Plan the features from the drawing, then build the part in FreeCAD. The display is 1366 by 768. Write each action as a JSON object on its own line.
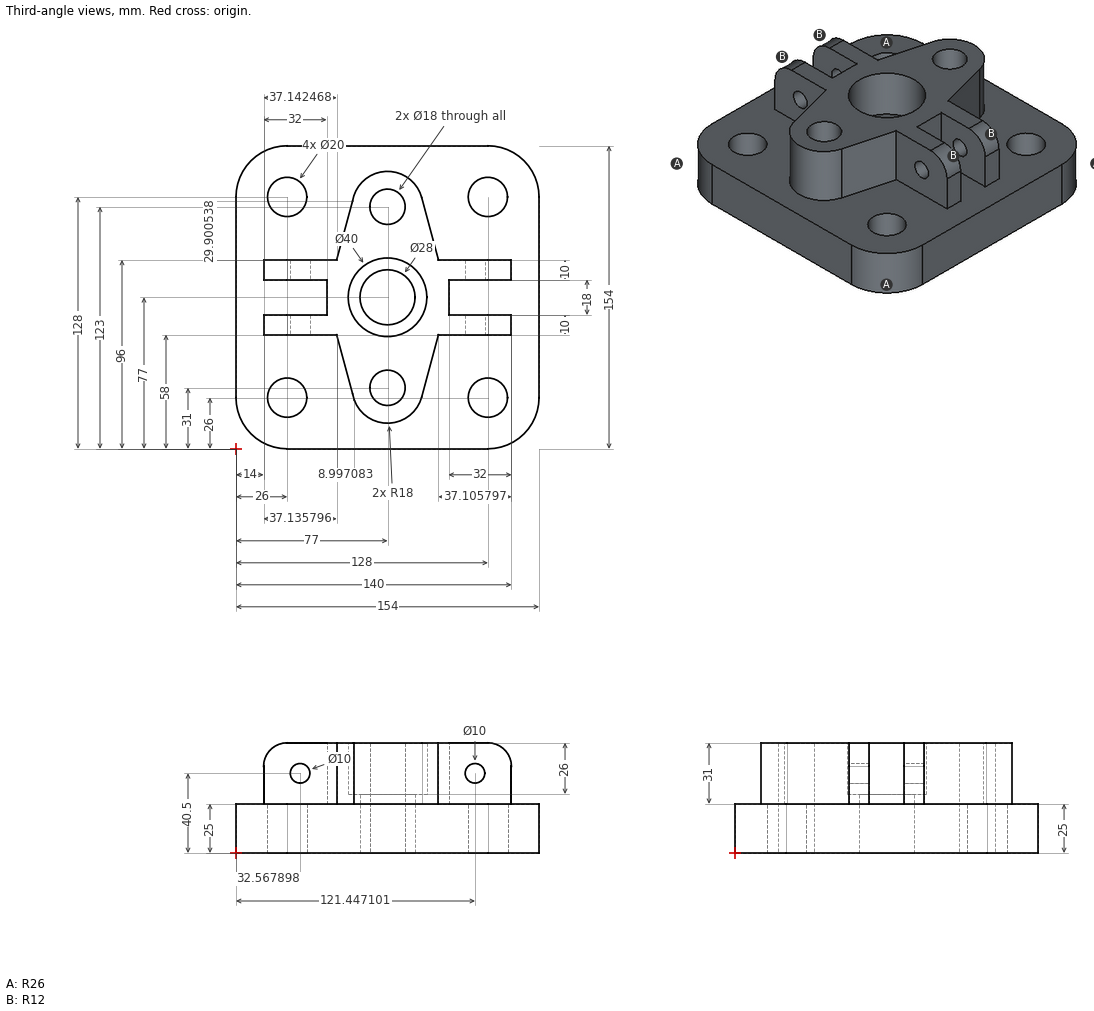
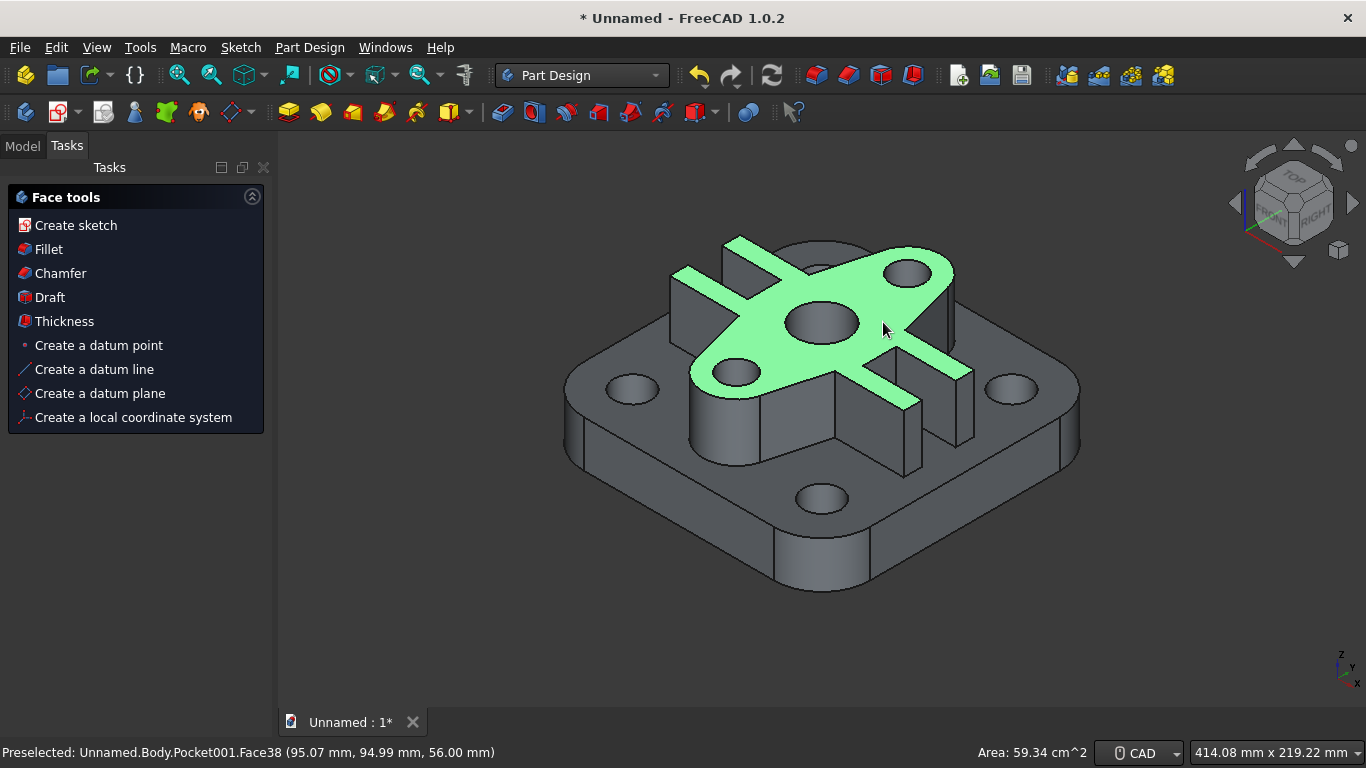
{"action": "left_click", "coordinate": [58, 112]}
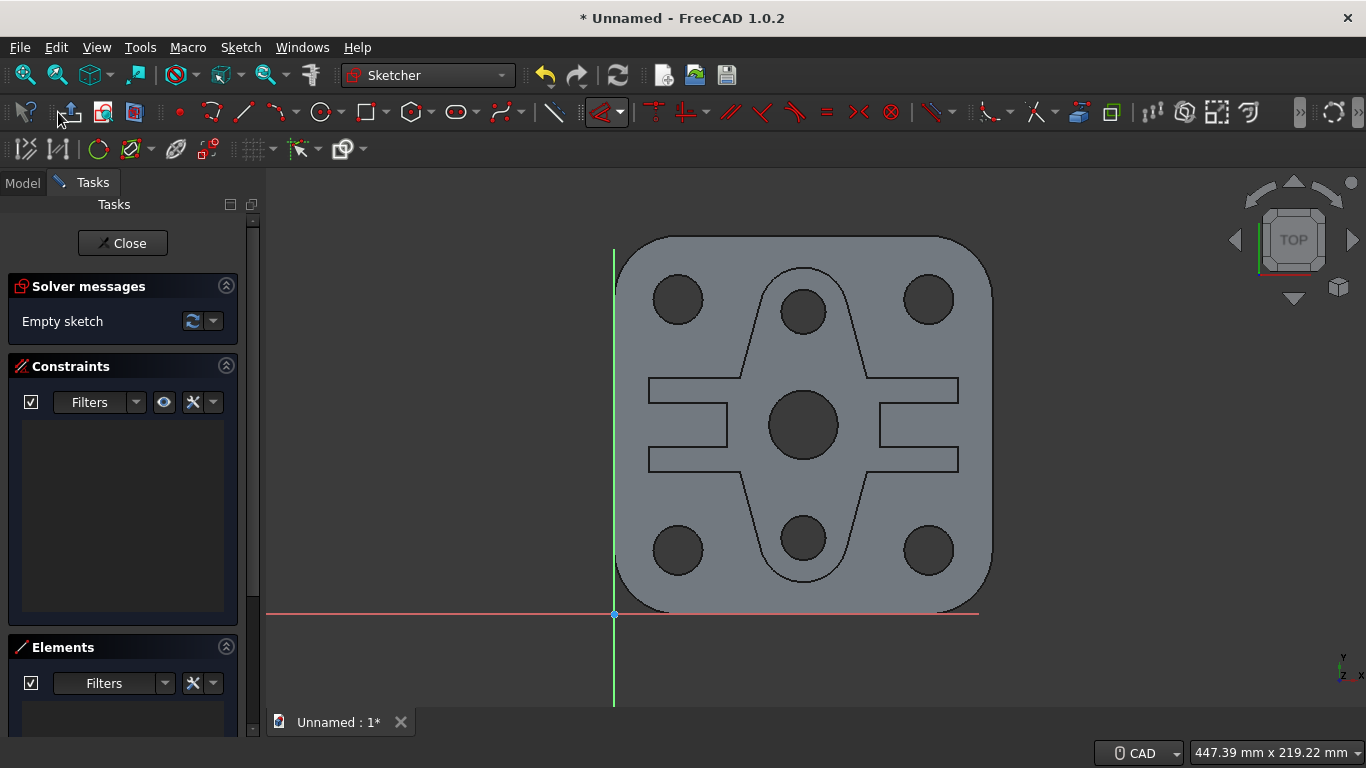
{"action": "scroll", "coordinate": [705, 612], "scroll_direction": "up", "scroll_amount": 2}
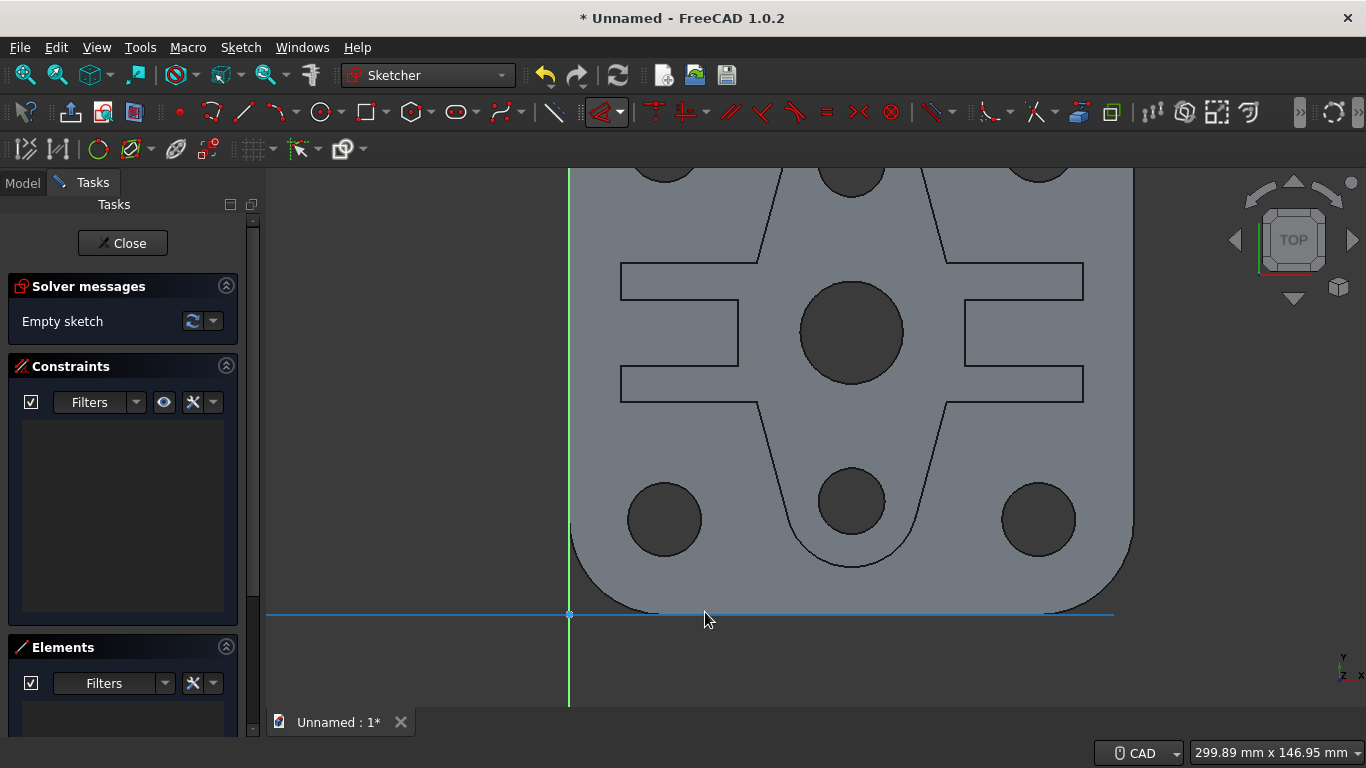
{"action": "left_click", "coordinate": [322, 112]}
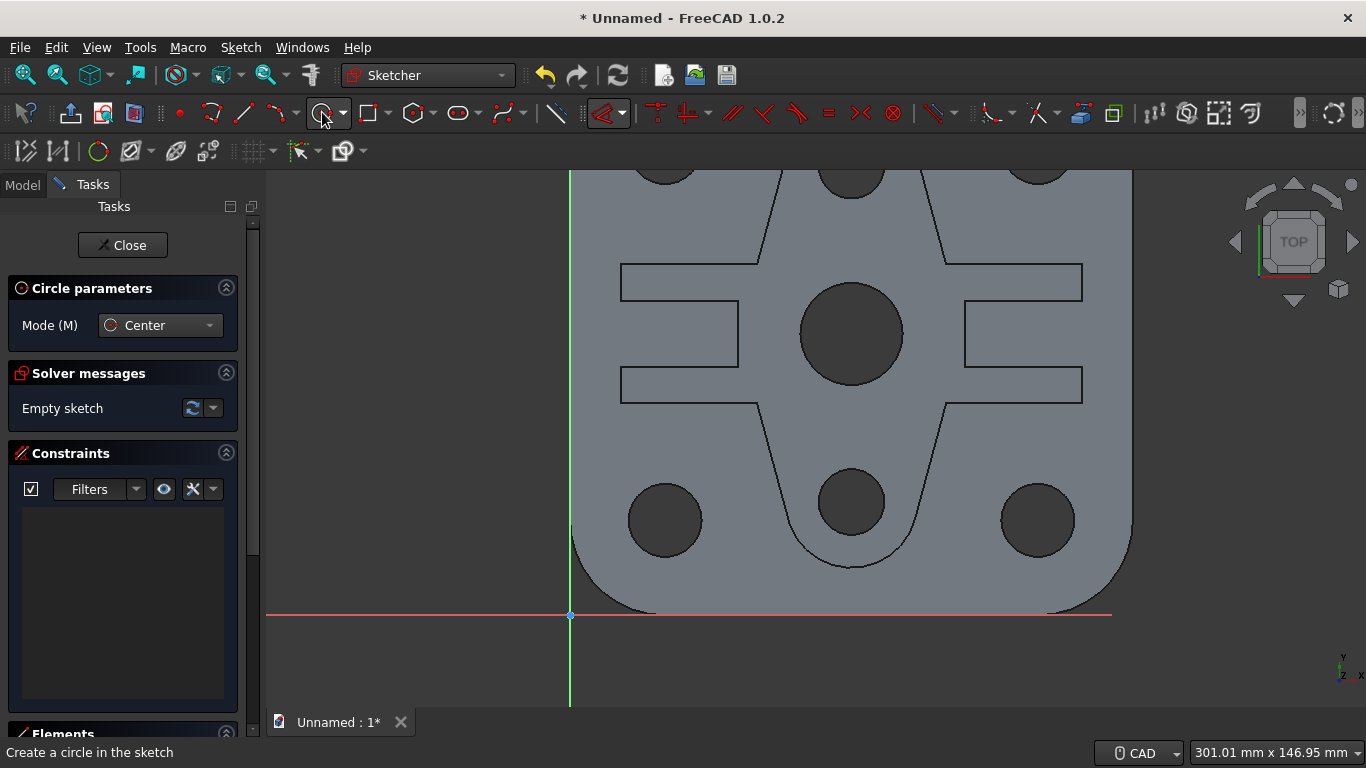
{"action": "left_click", "coordinate": [852, 334]}
{"action": "left_click", "coordinate": [903, 282]}
{"action": "key", "text": "Escape"}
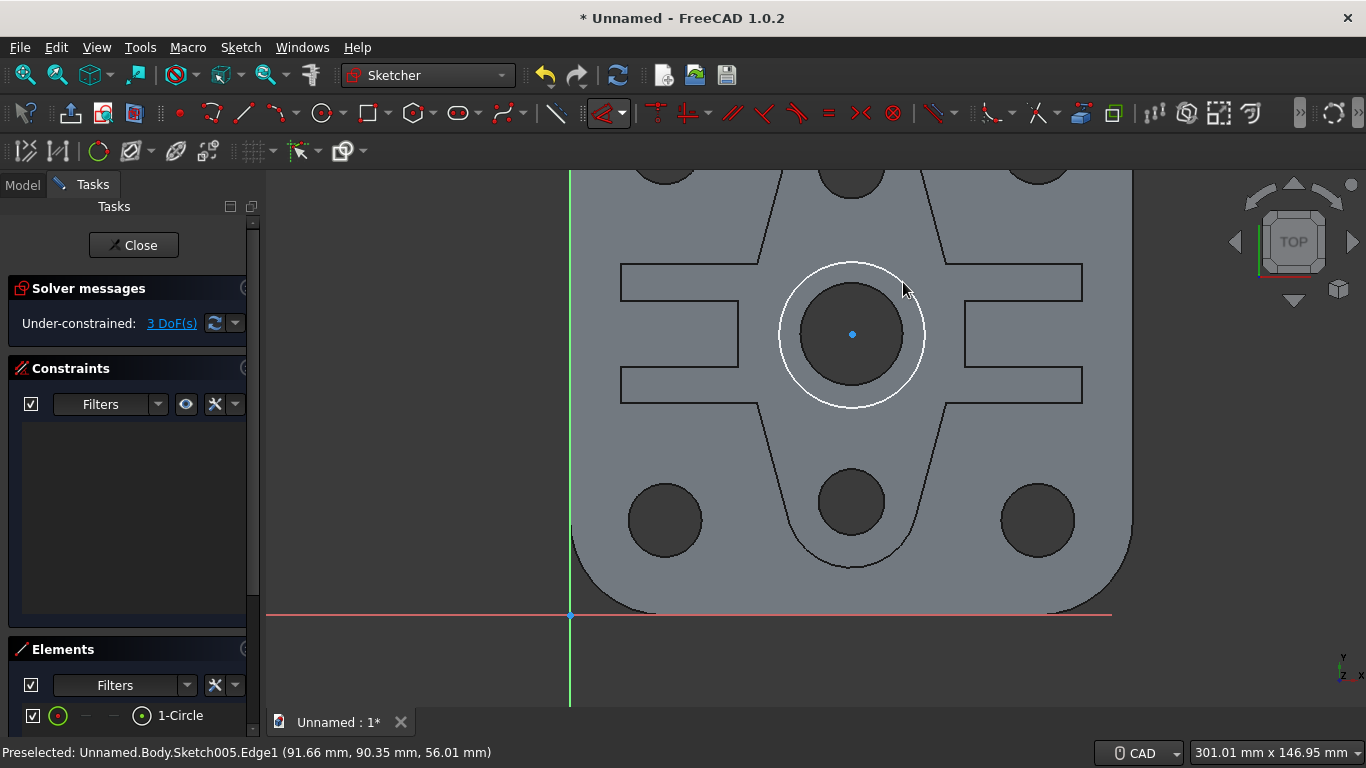
{"action": "left_click", "coordinate": [903, 283]}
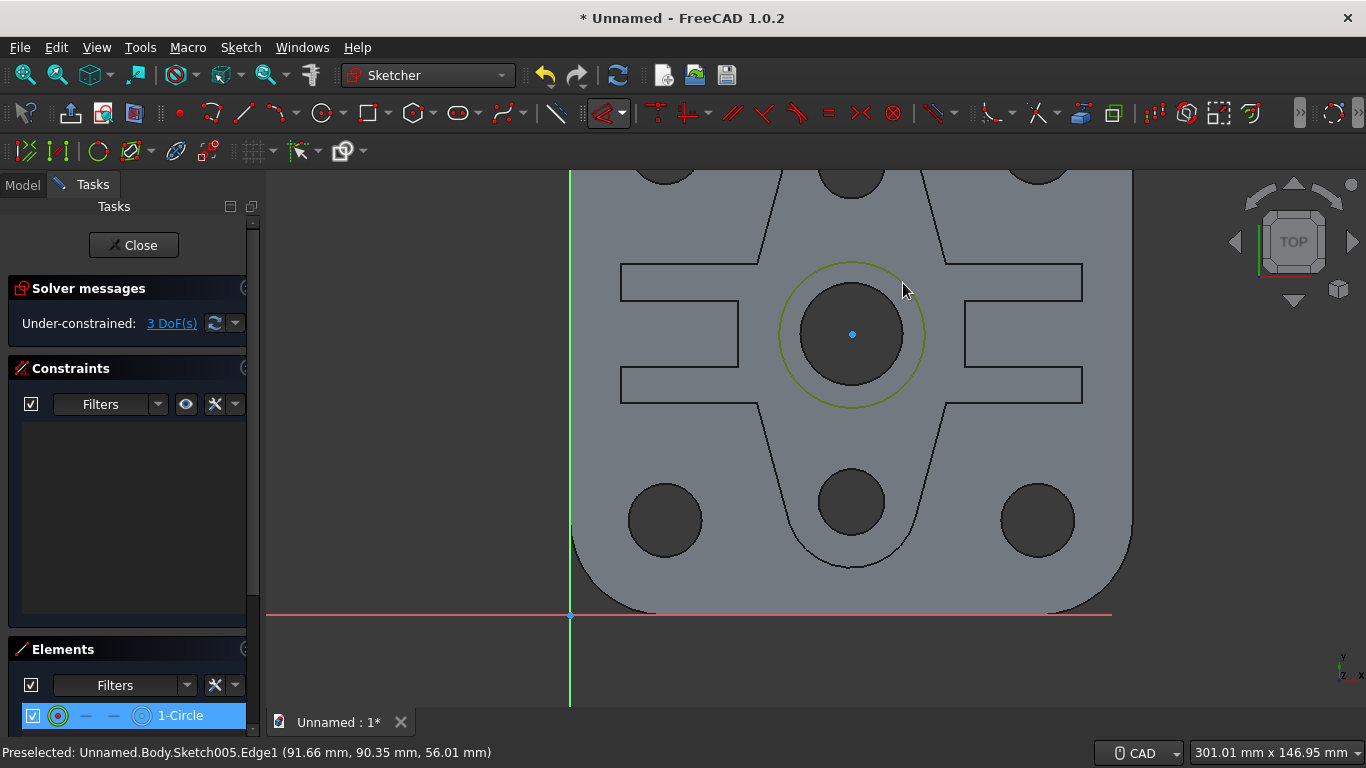
{"action": "left_click", "coordinate": [624, 114]}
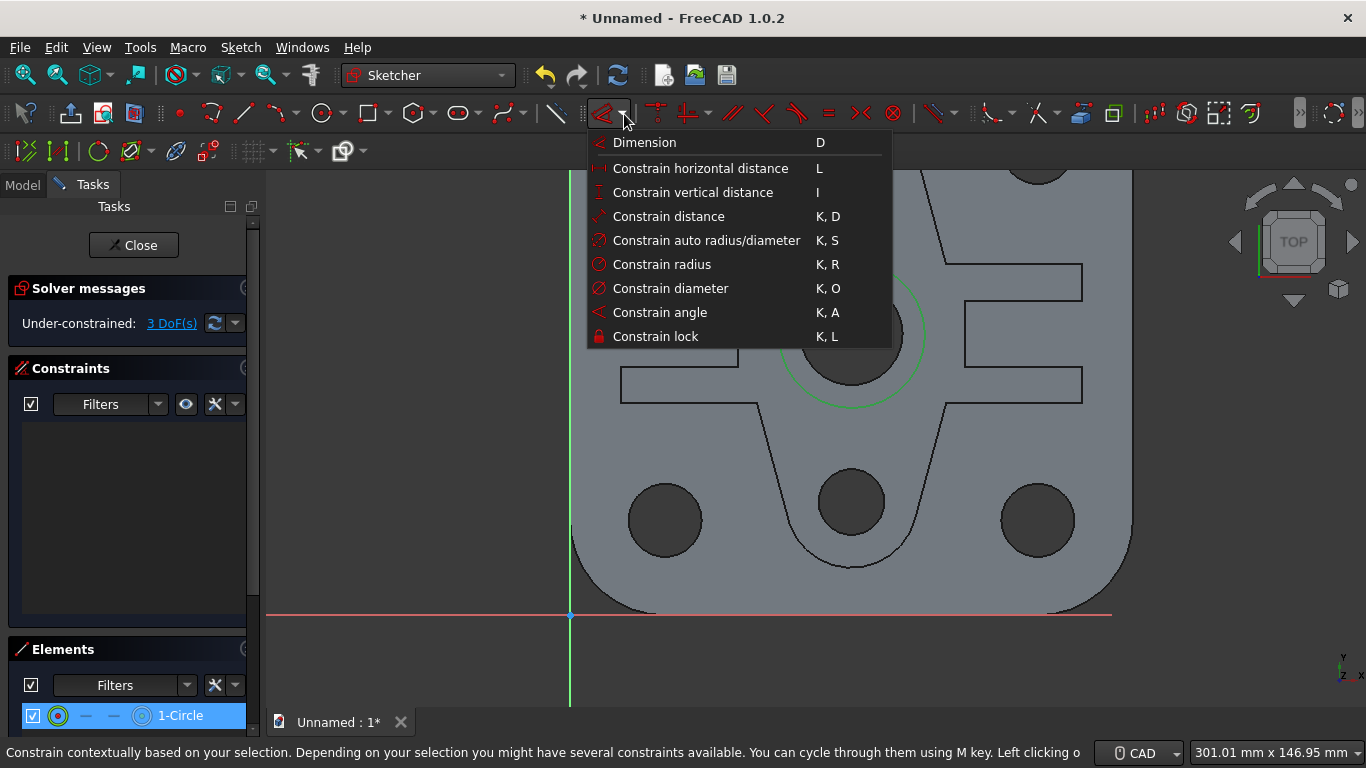
{"action": "left_click", "coordinate": [740, 288]}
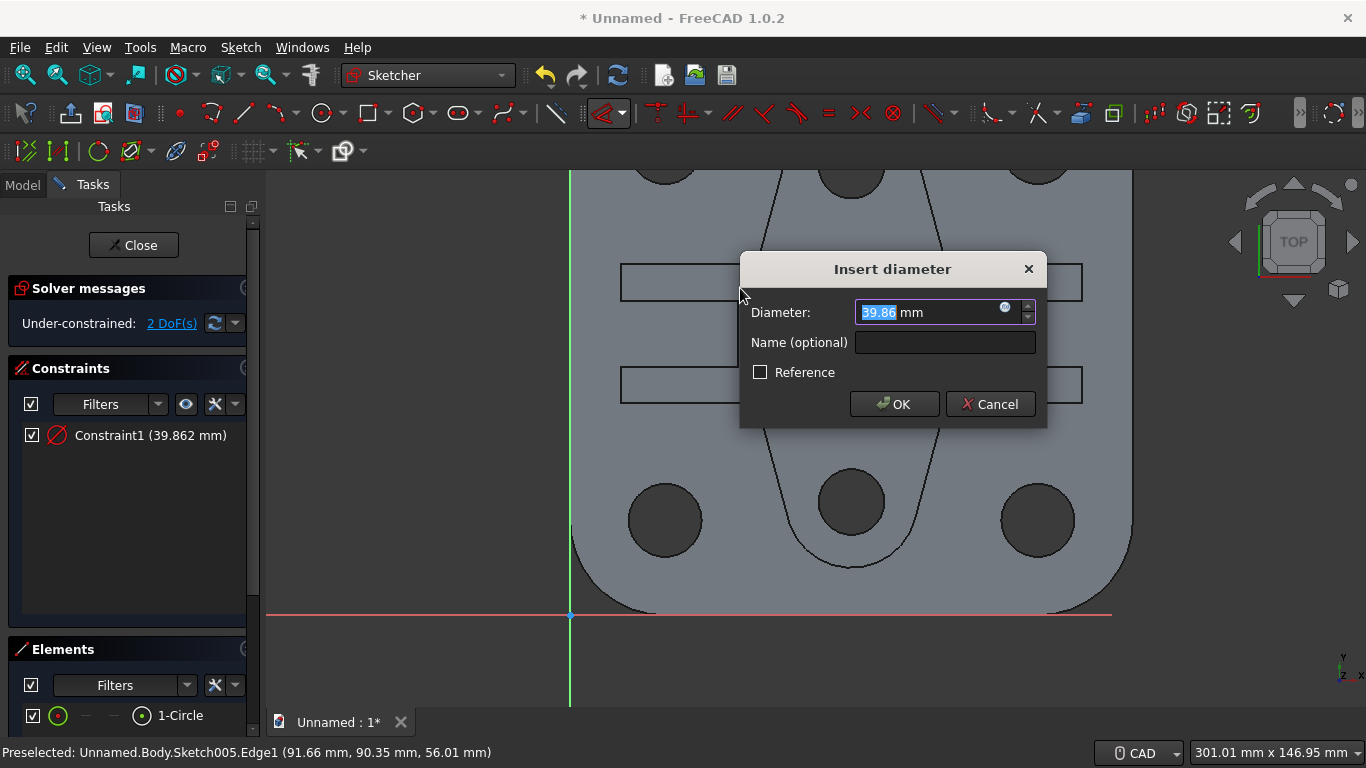
{"action": "type", "text": "40"}
{"action": "key", "text": "Return"}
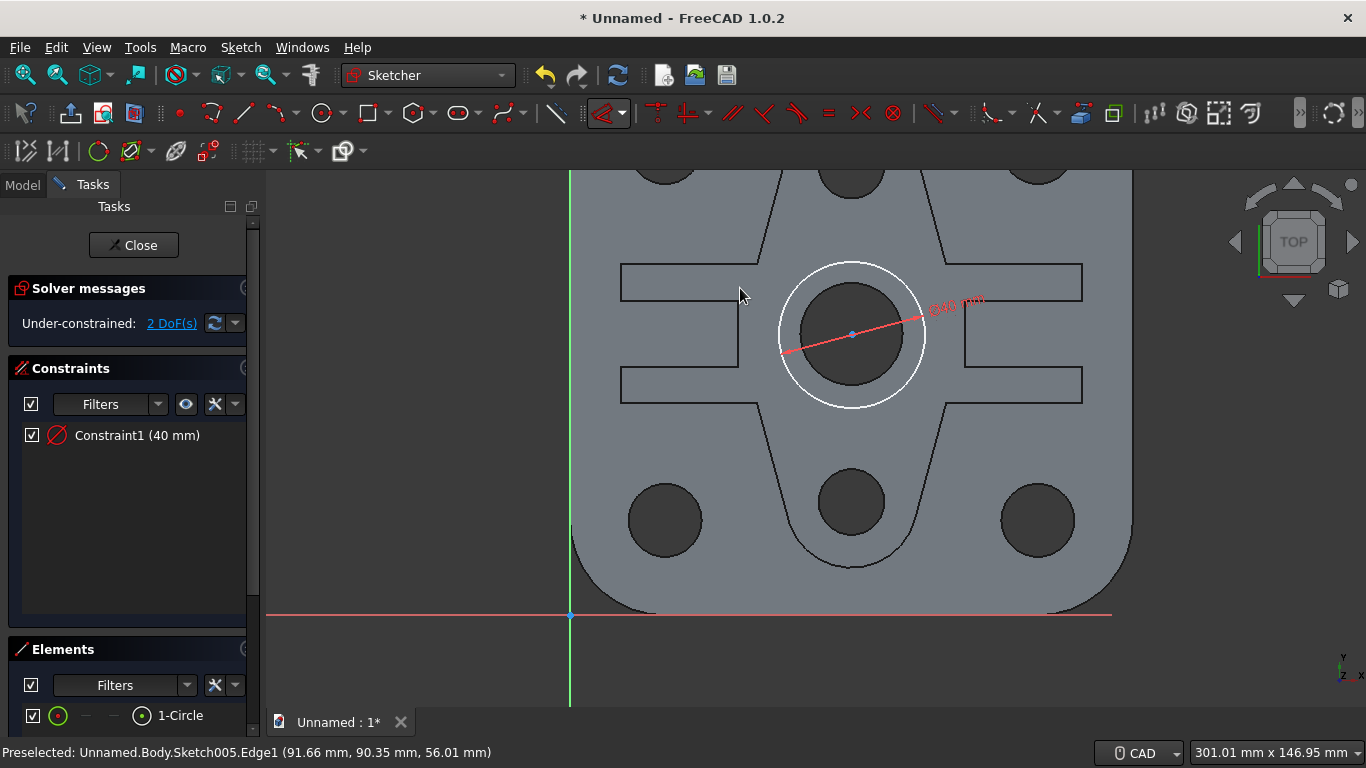
{"action": "left_click", "coordinate": [852, 335]}